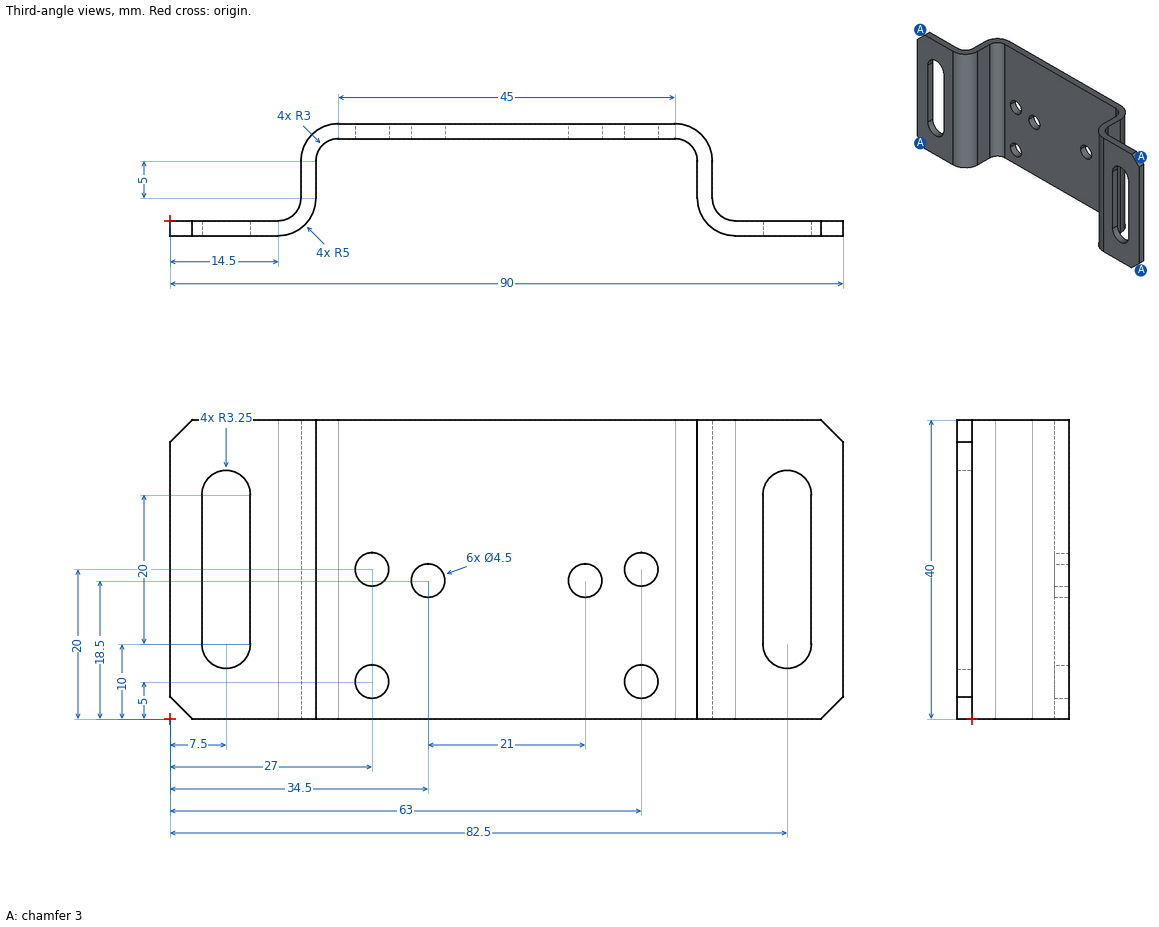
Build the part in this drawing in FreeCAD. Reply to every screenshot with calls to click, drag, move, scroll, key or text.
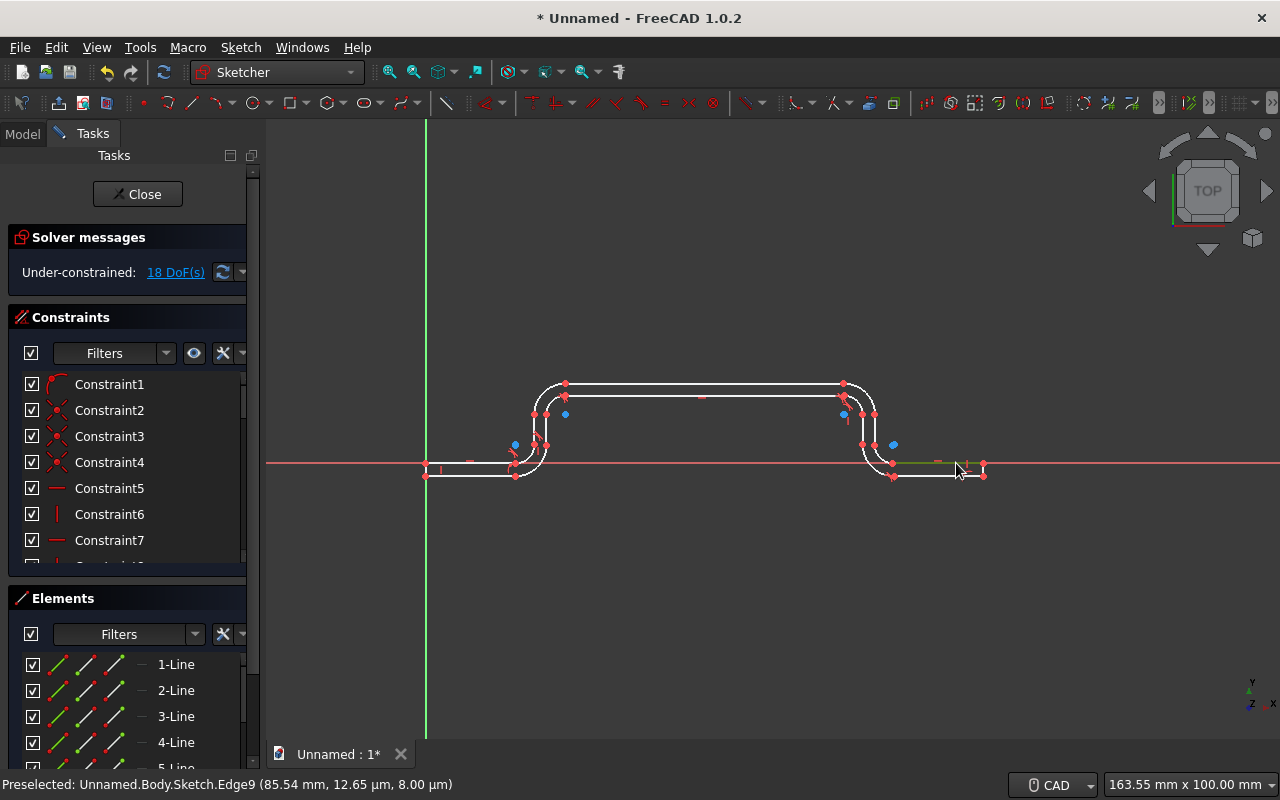
click(574, 104)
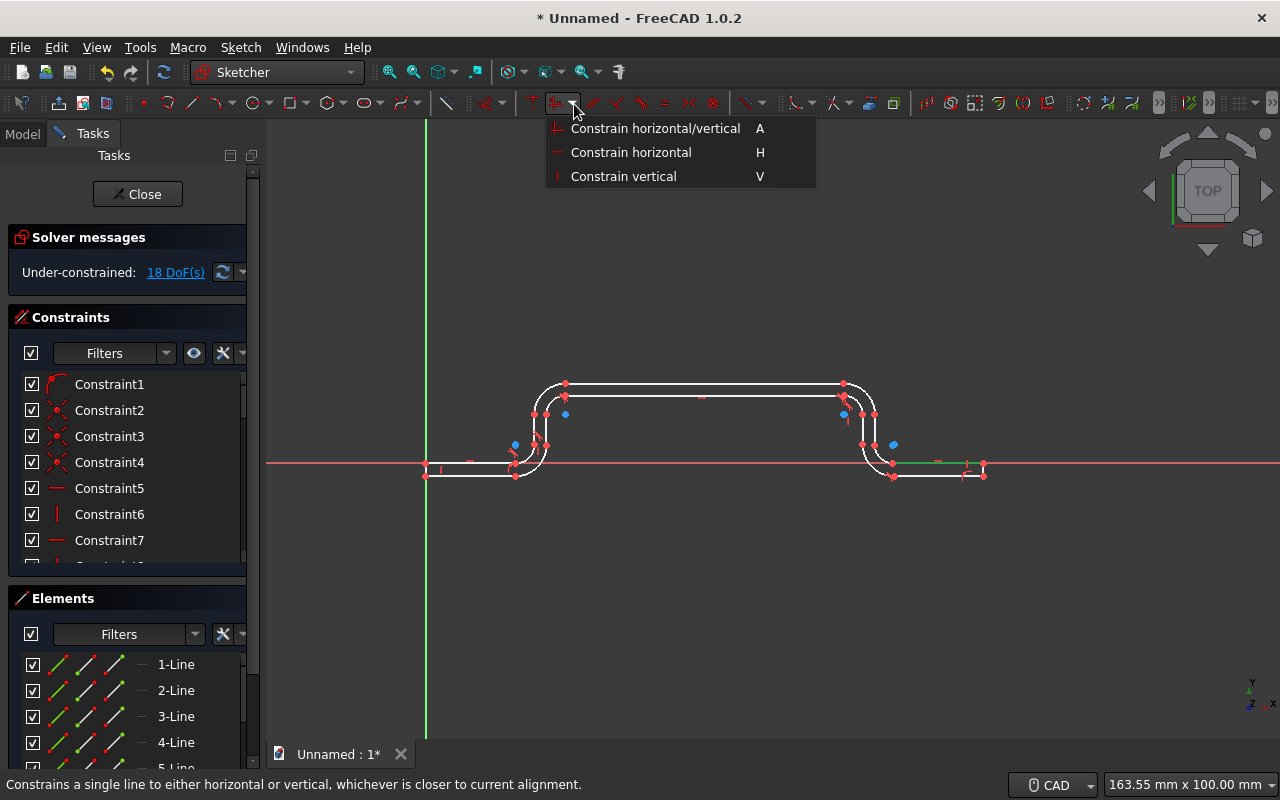
click(681, 152)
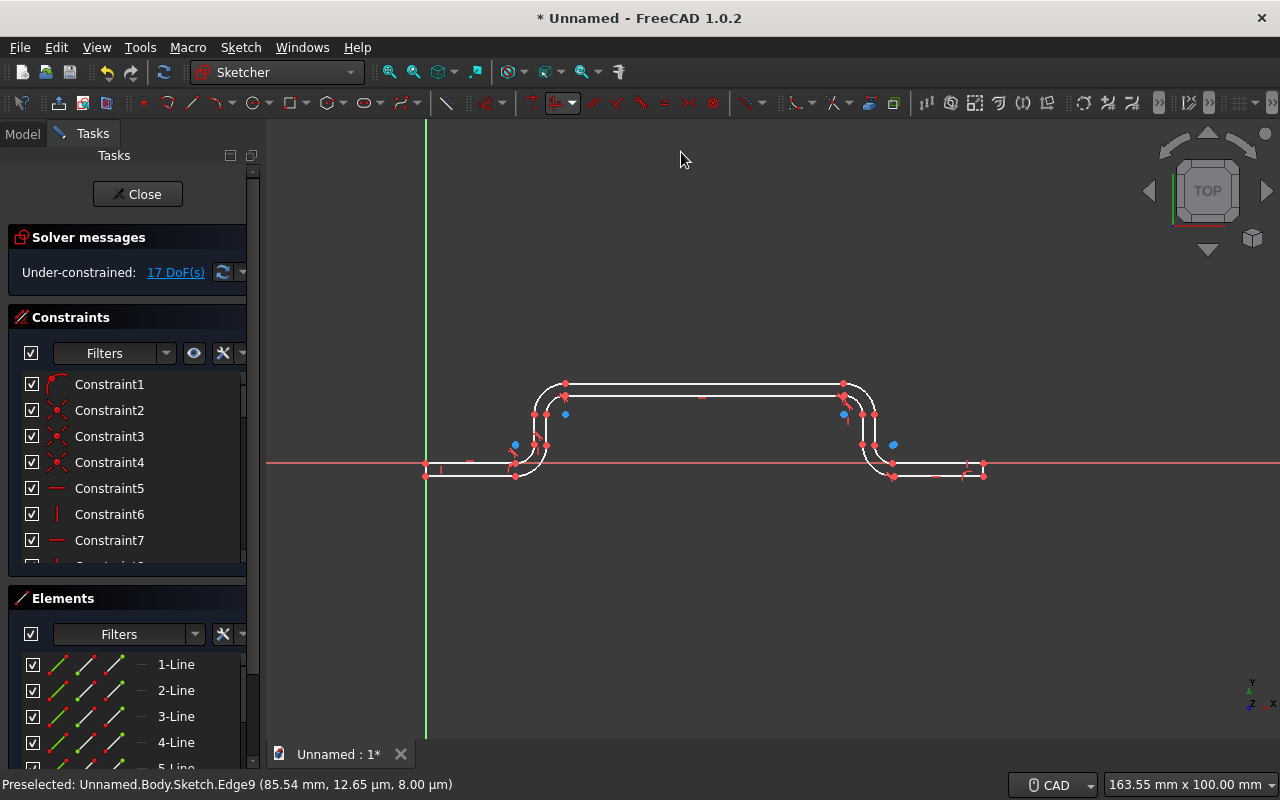
scroll(880, 473, up, 2)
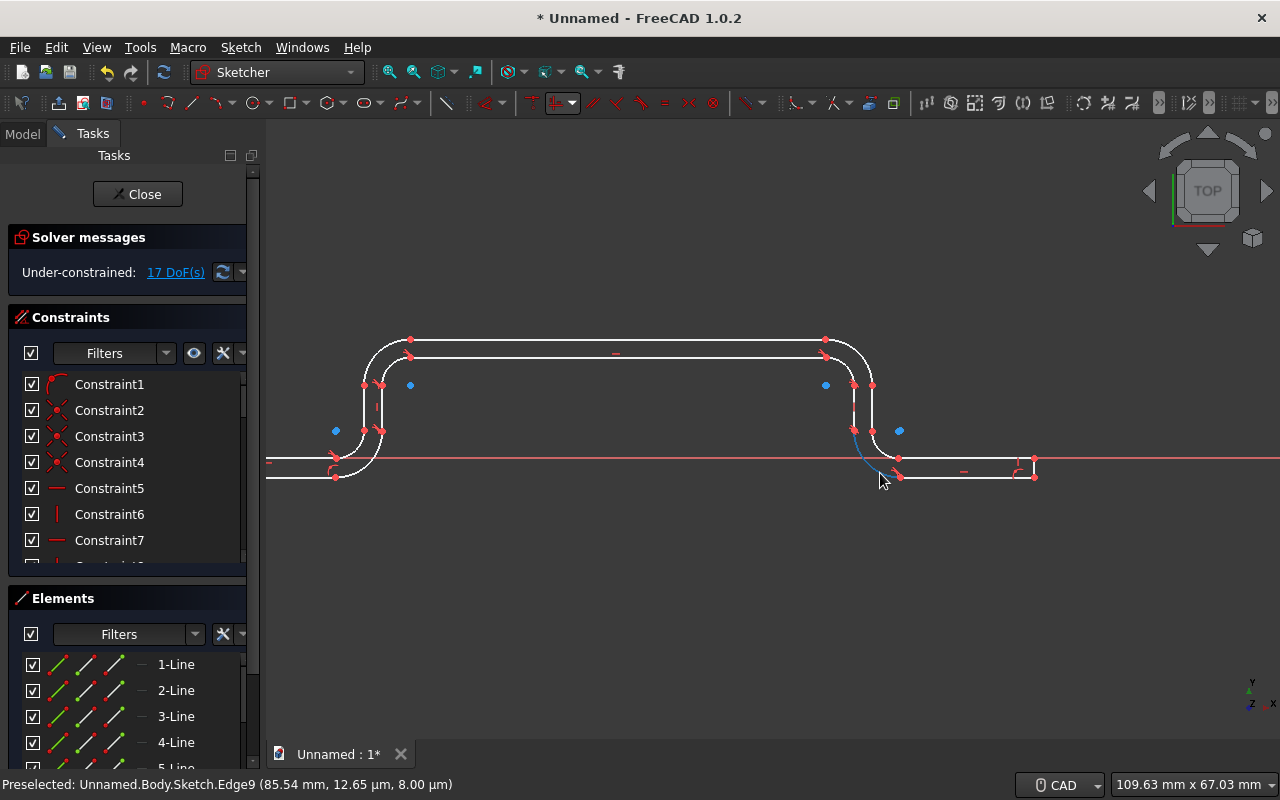
click(880, 472)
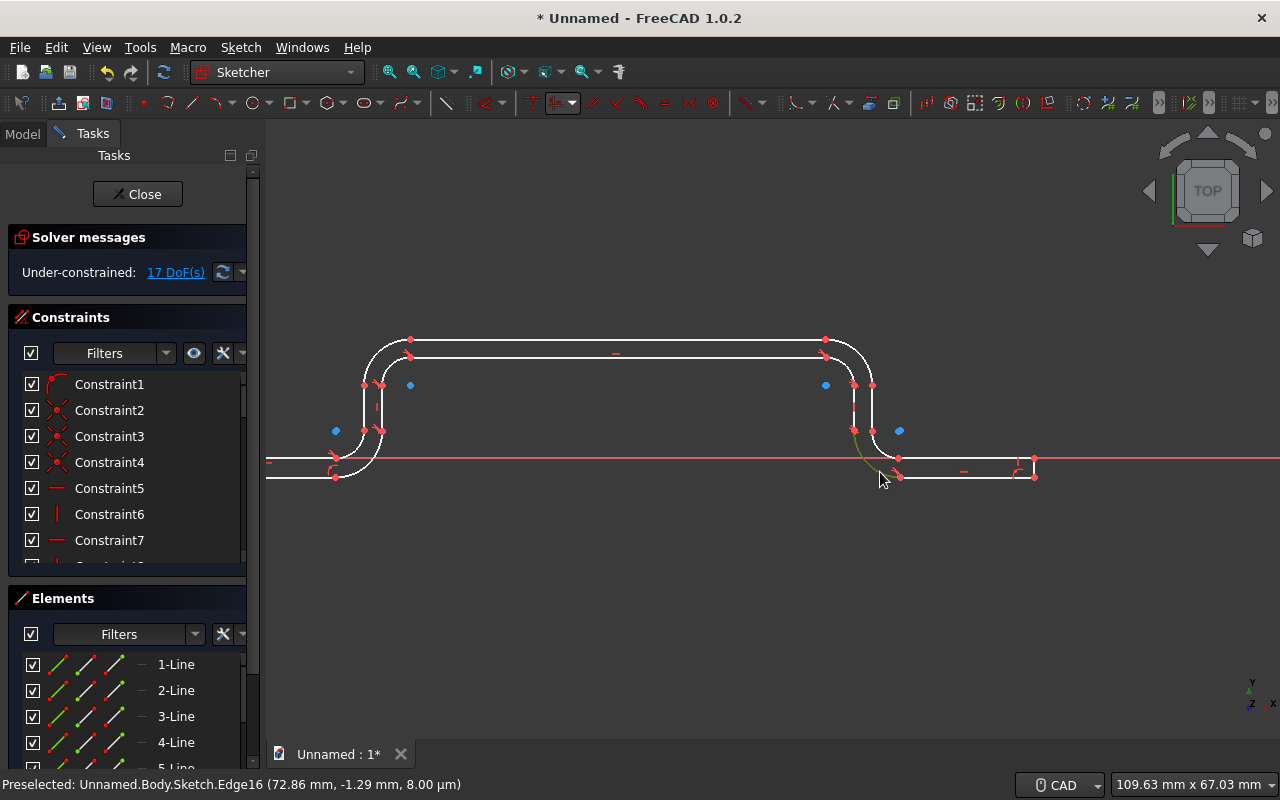
click(875, 444)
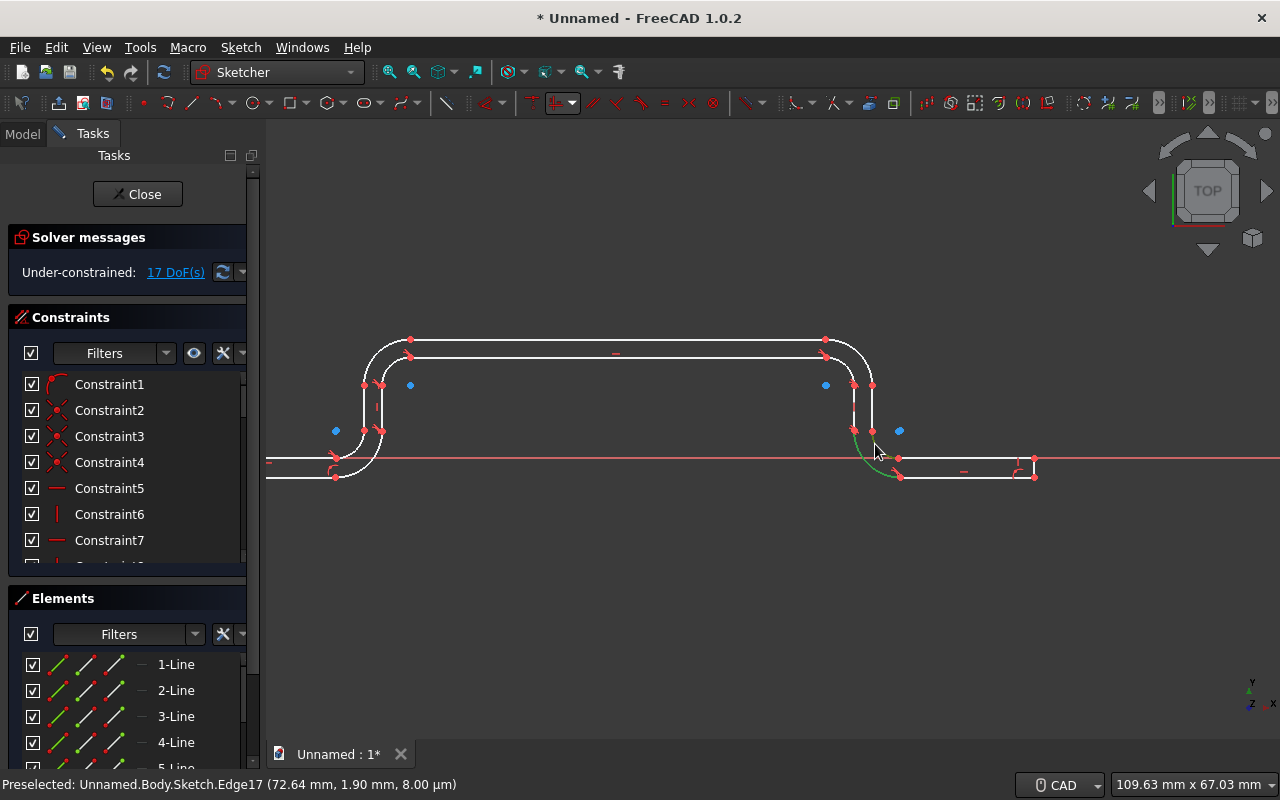
key(c)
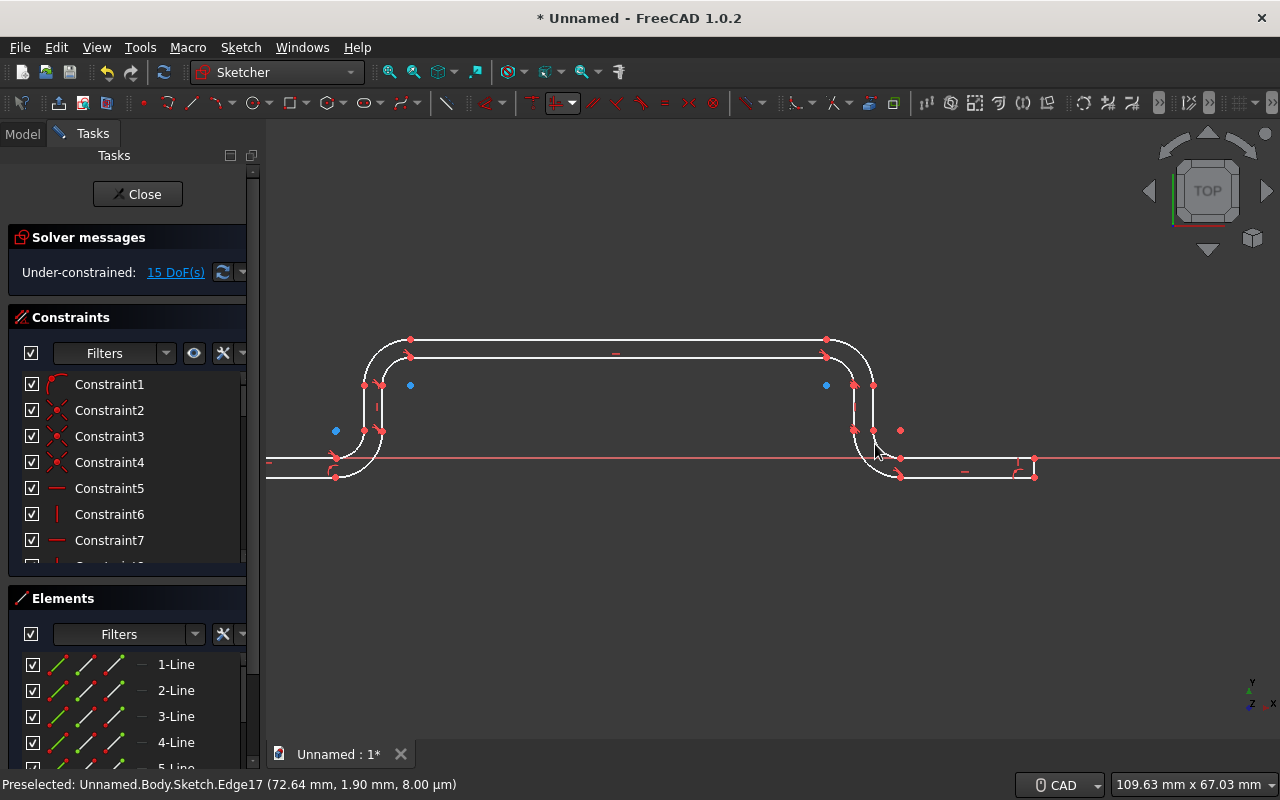
click(851, 373)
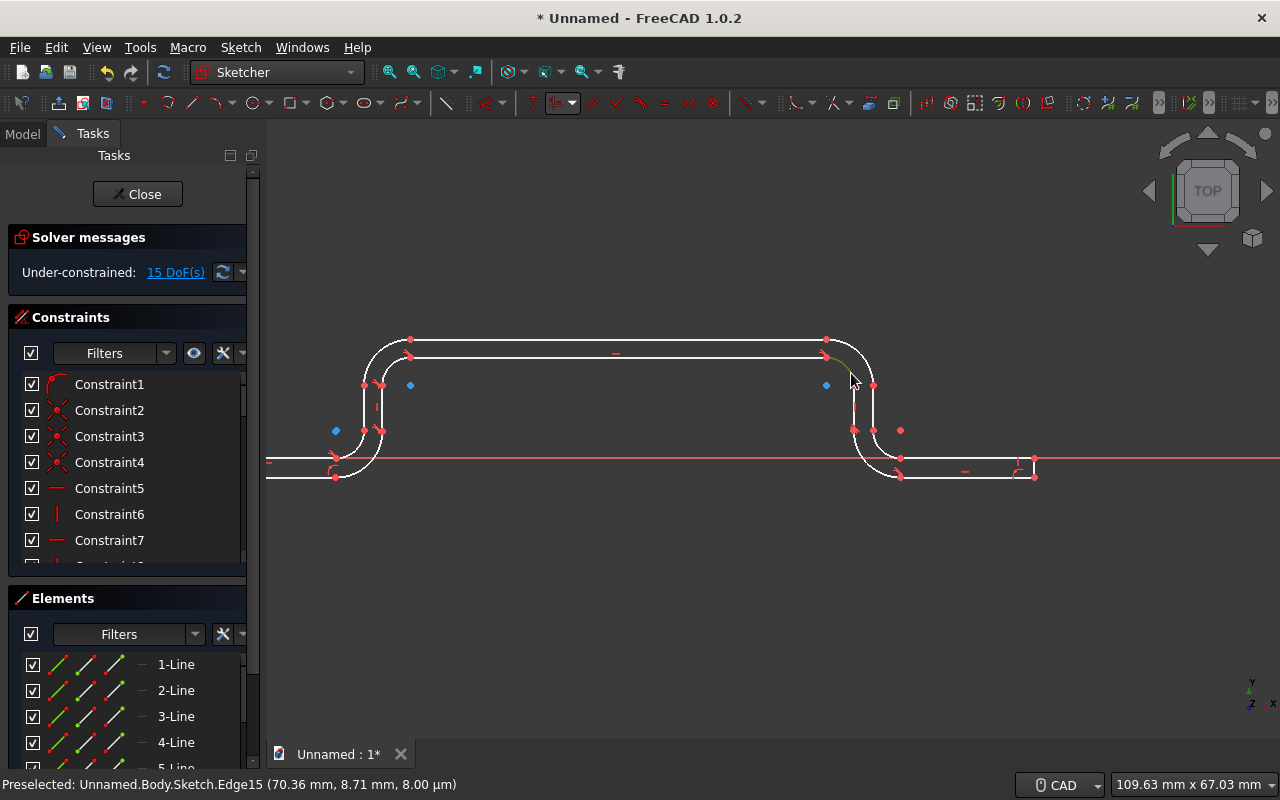
click(868, 365)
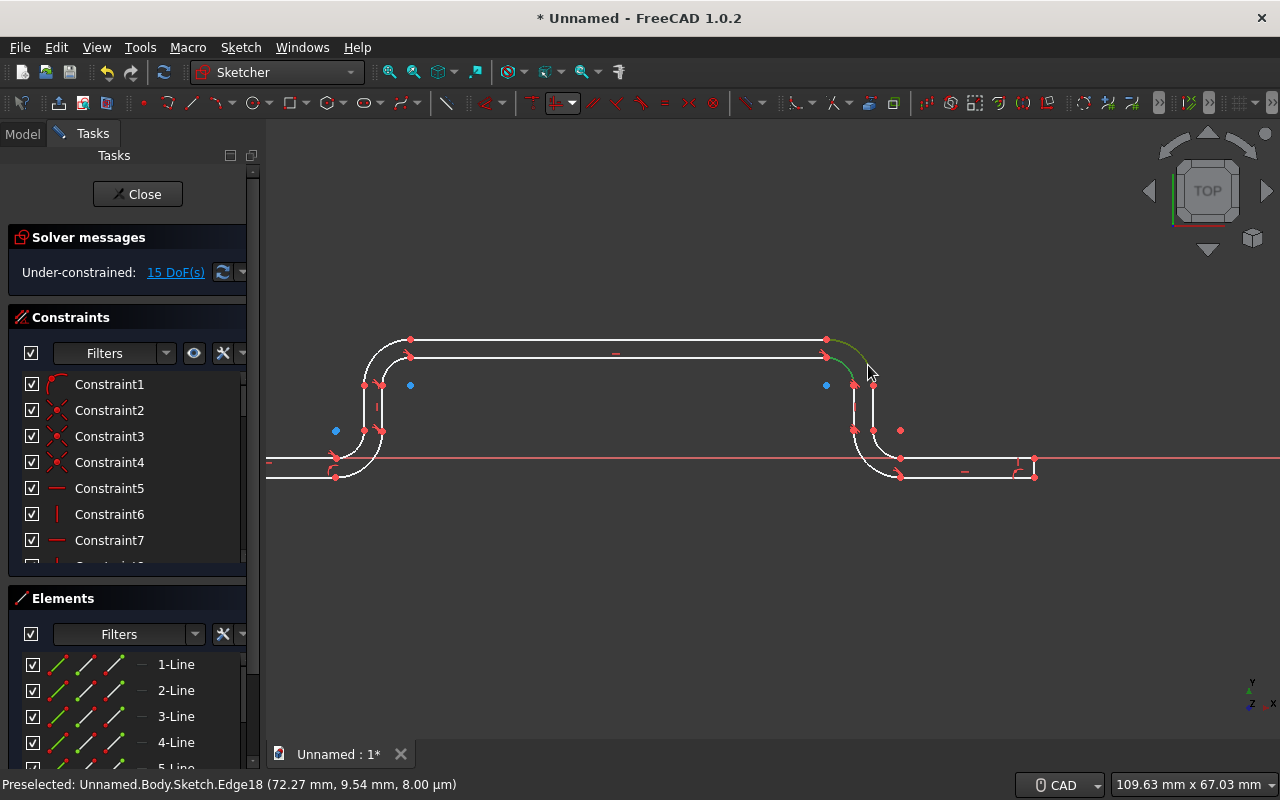
key(c)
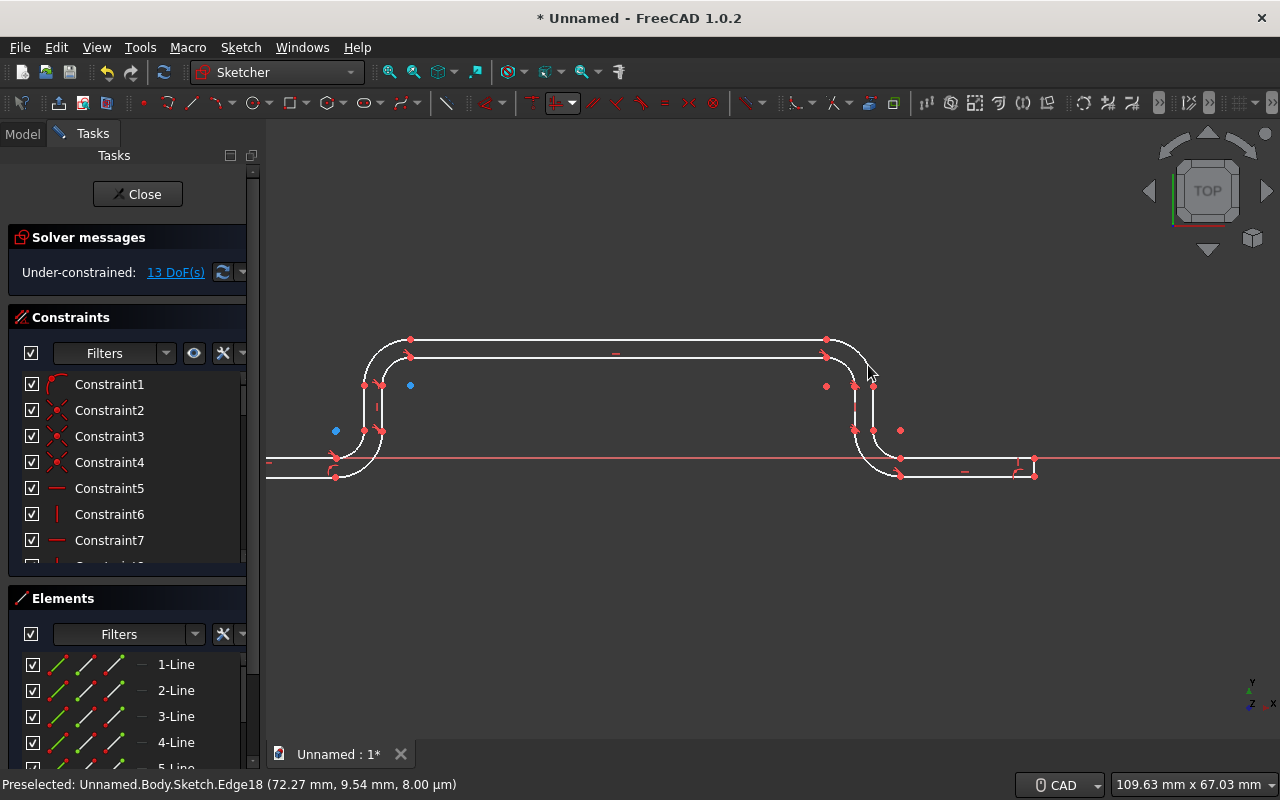
click(397, 361)